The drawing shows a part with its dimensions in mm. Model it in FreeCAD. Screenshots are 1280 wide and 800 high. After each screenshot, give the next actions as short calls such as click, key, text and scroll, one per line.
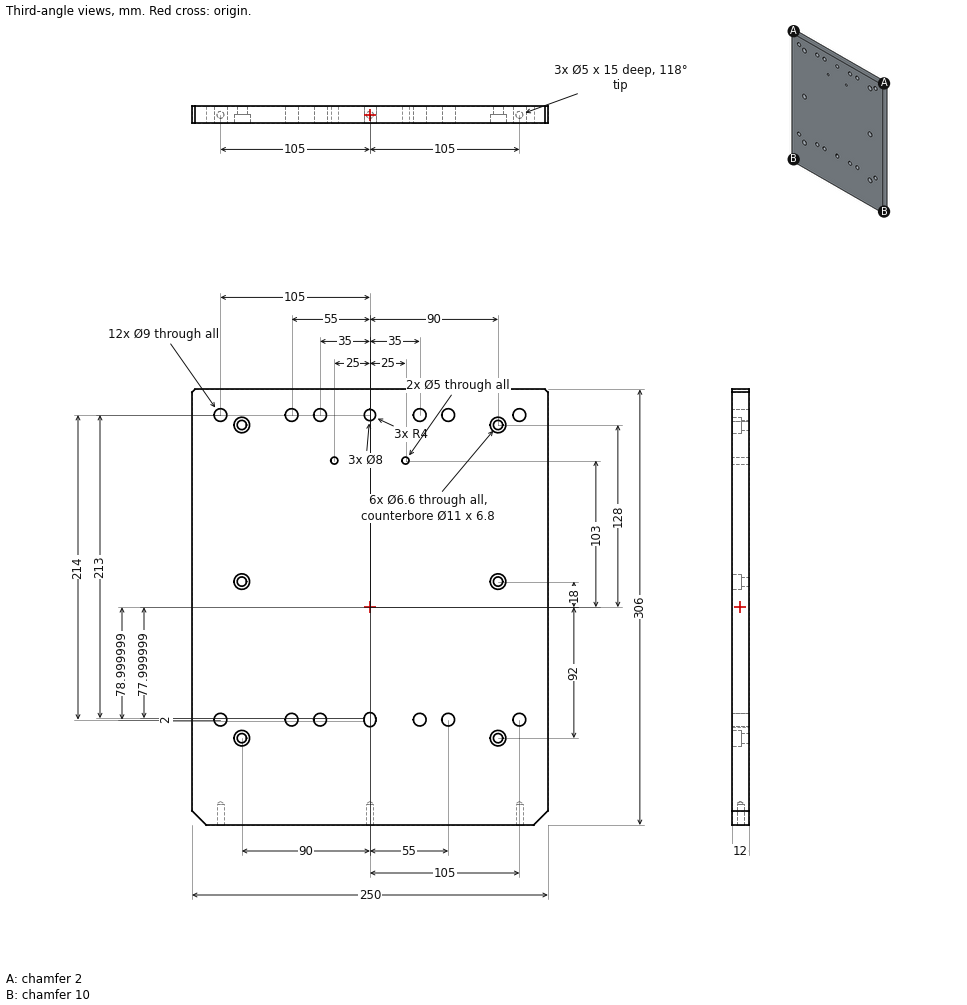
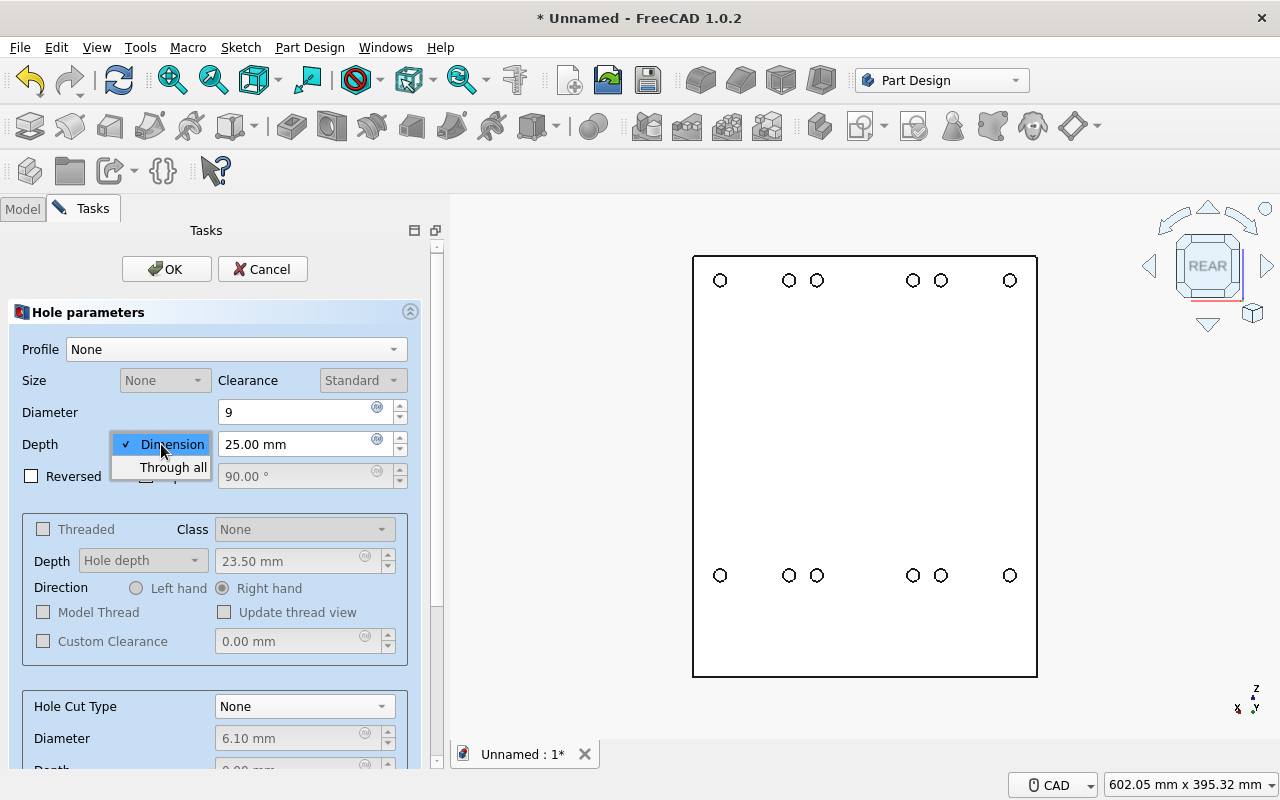
click(160, 468)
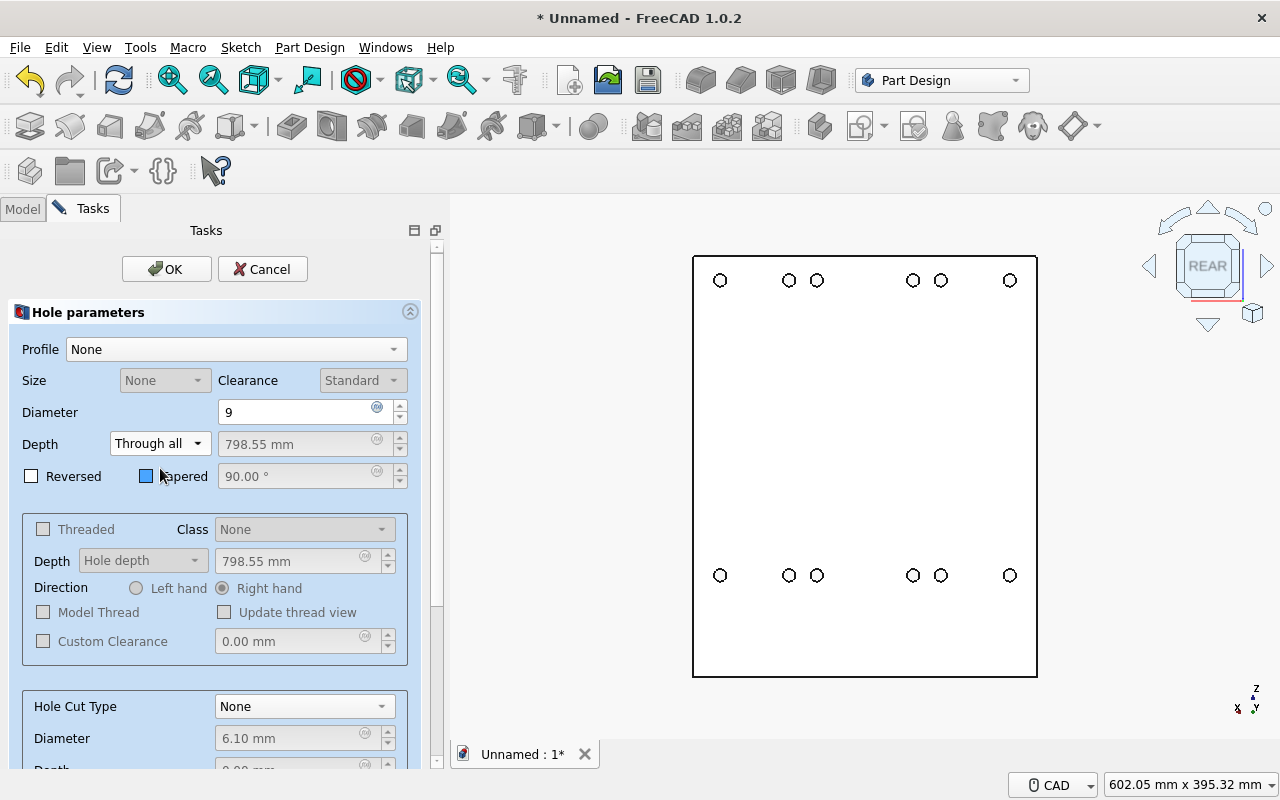
click(167, 269)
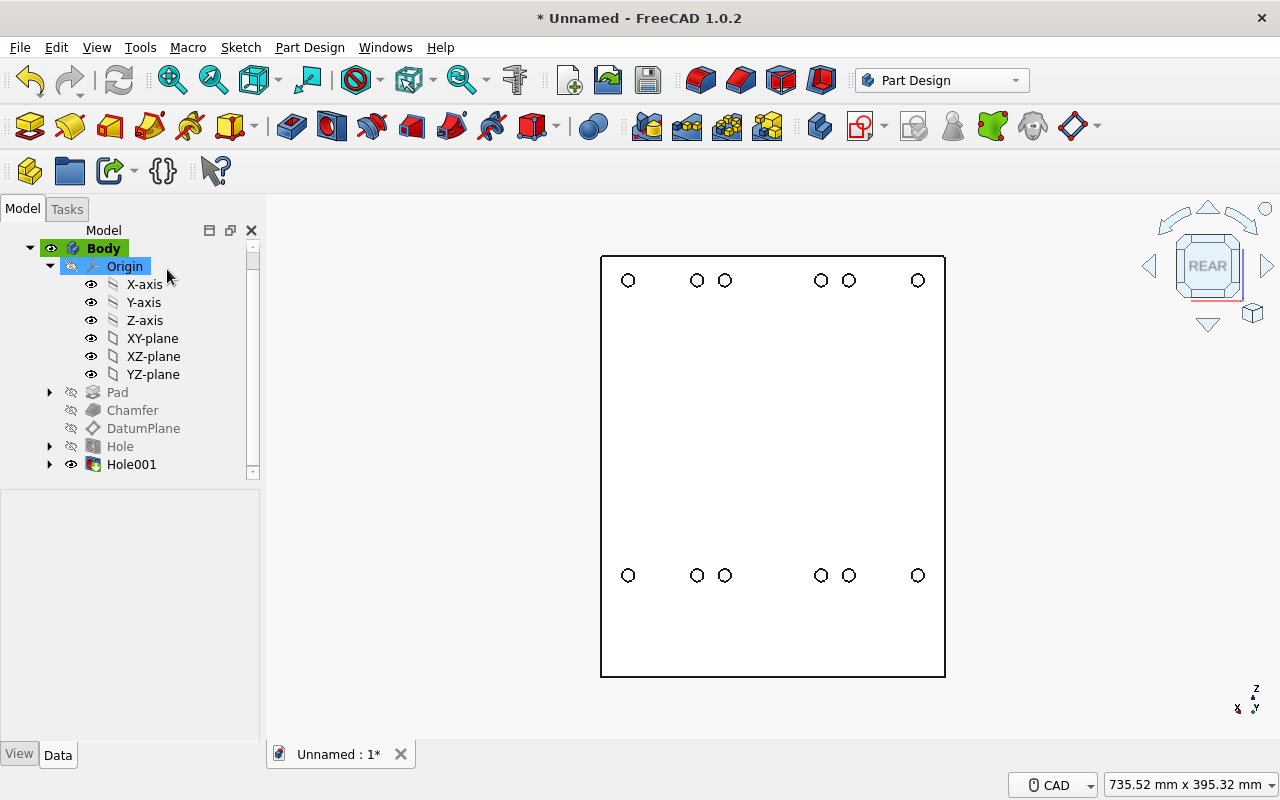
key(0)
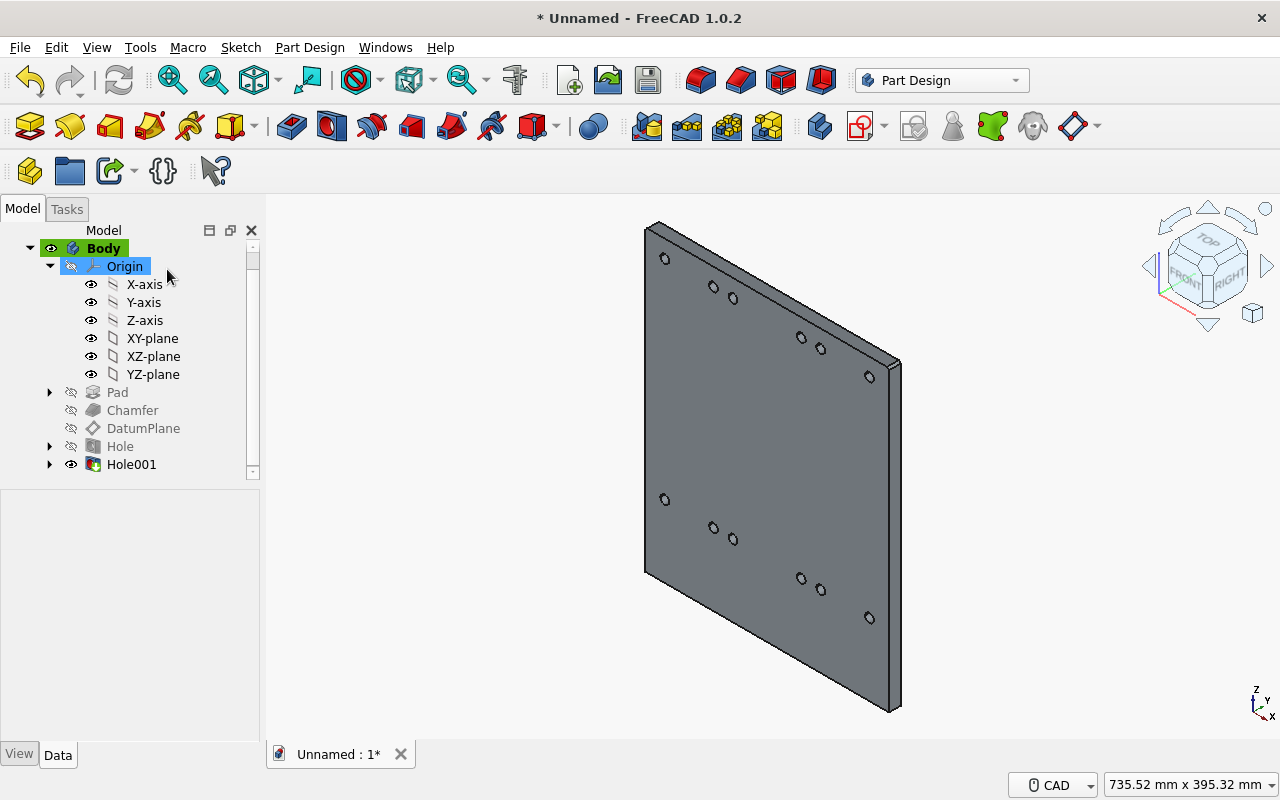
click(767, 420)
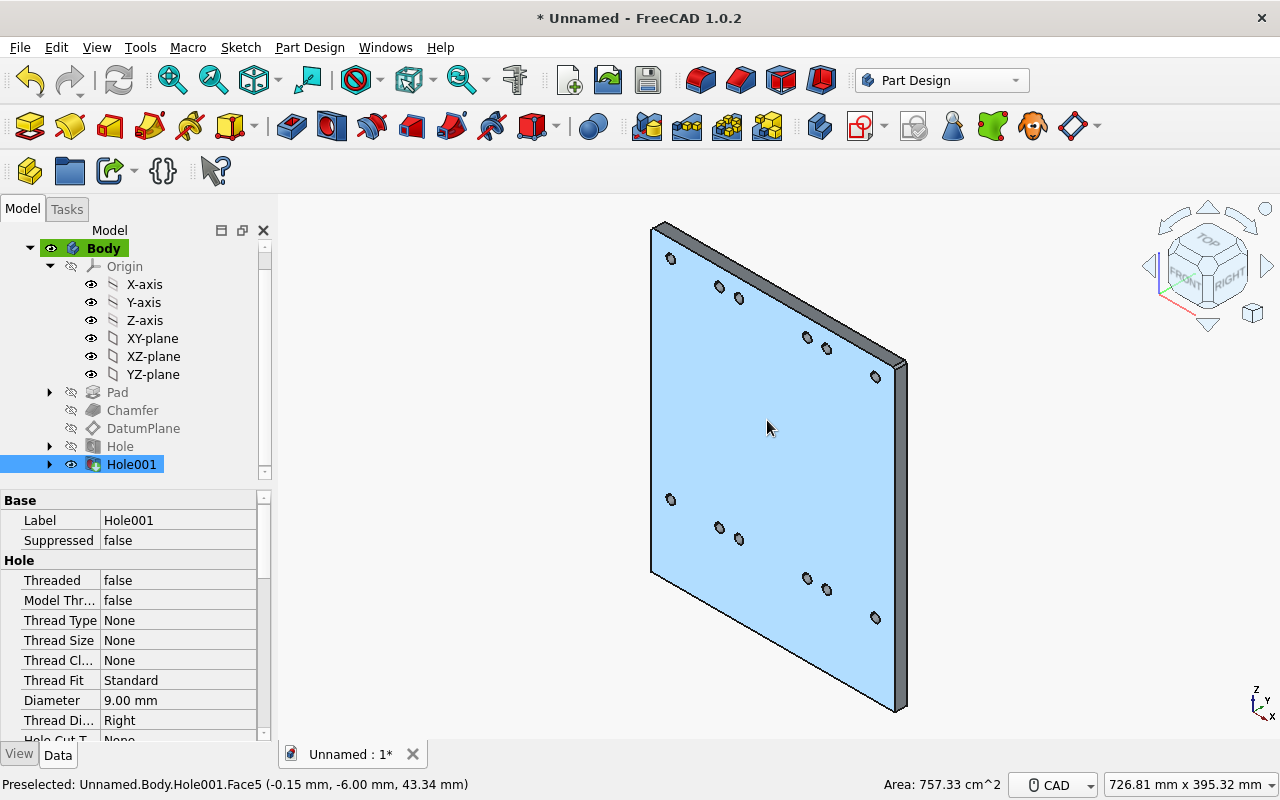
click(860, 126)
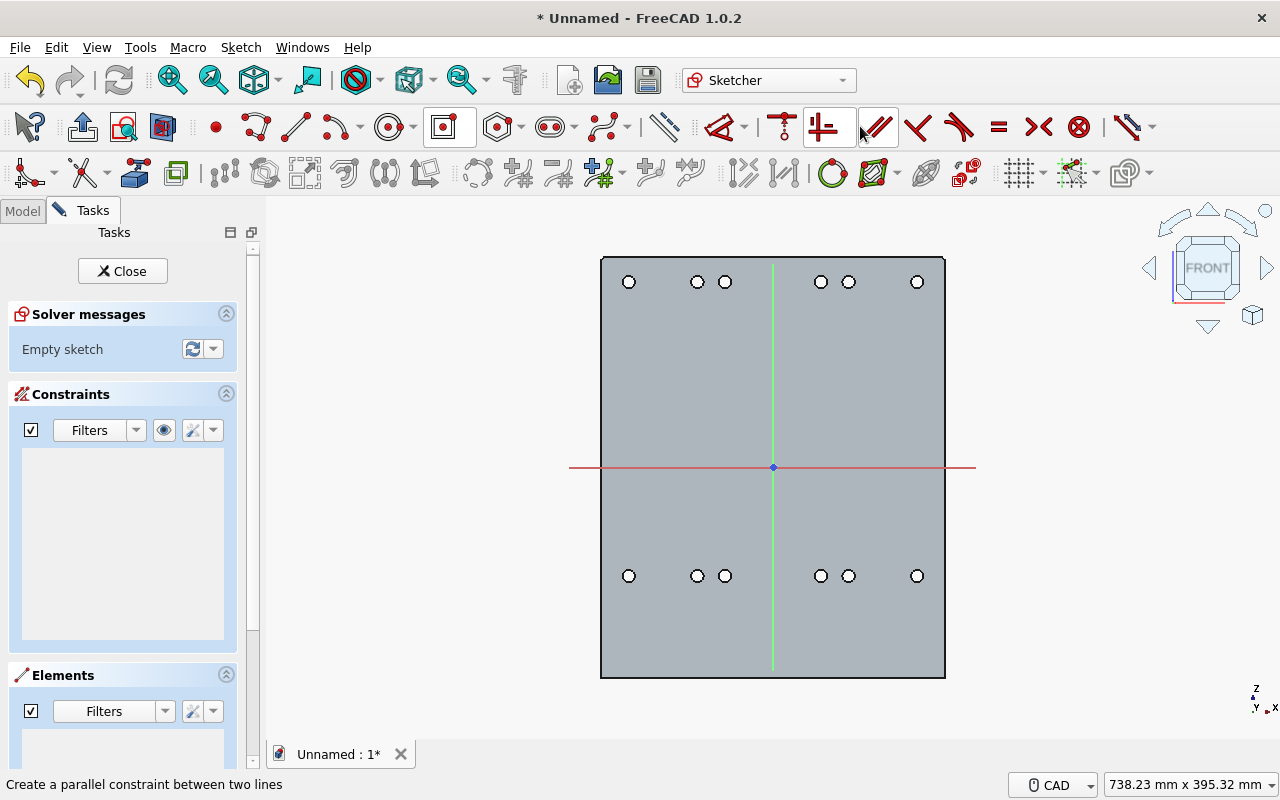
click(390, 128)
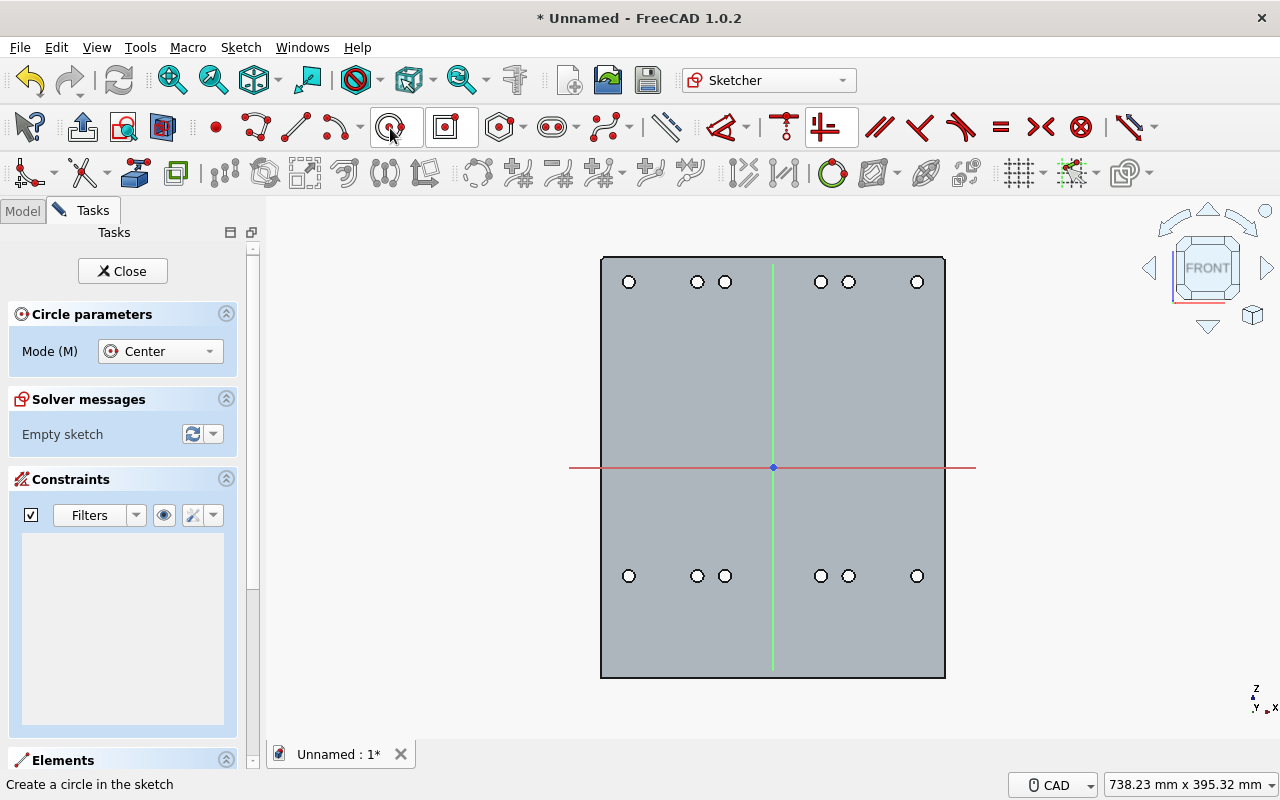
scroll(897, 292, up, 9)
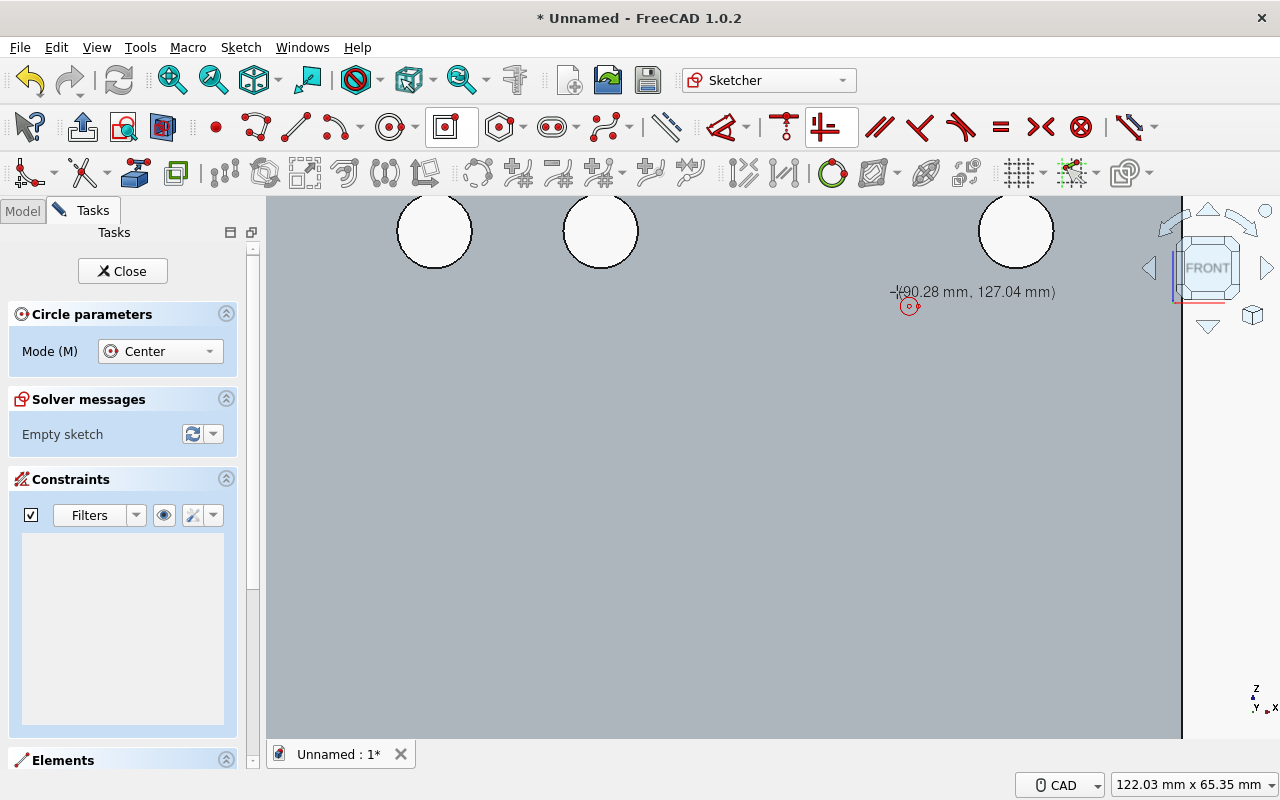
scroll(816, 322, down, 9)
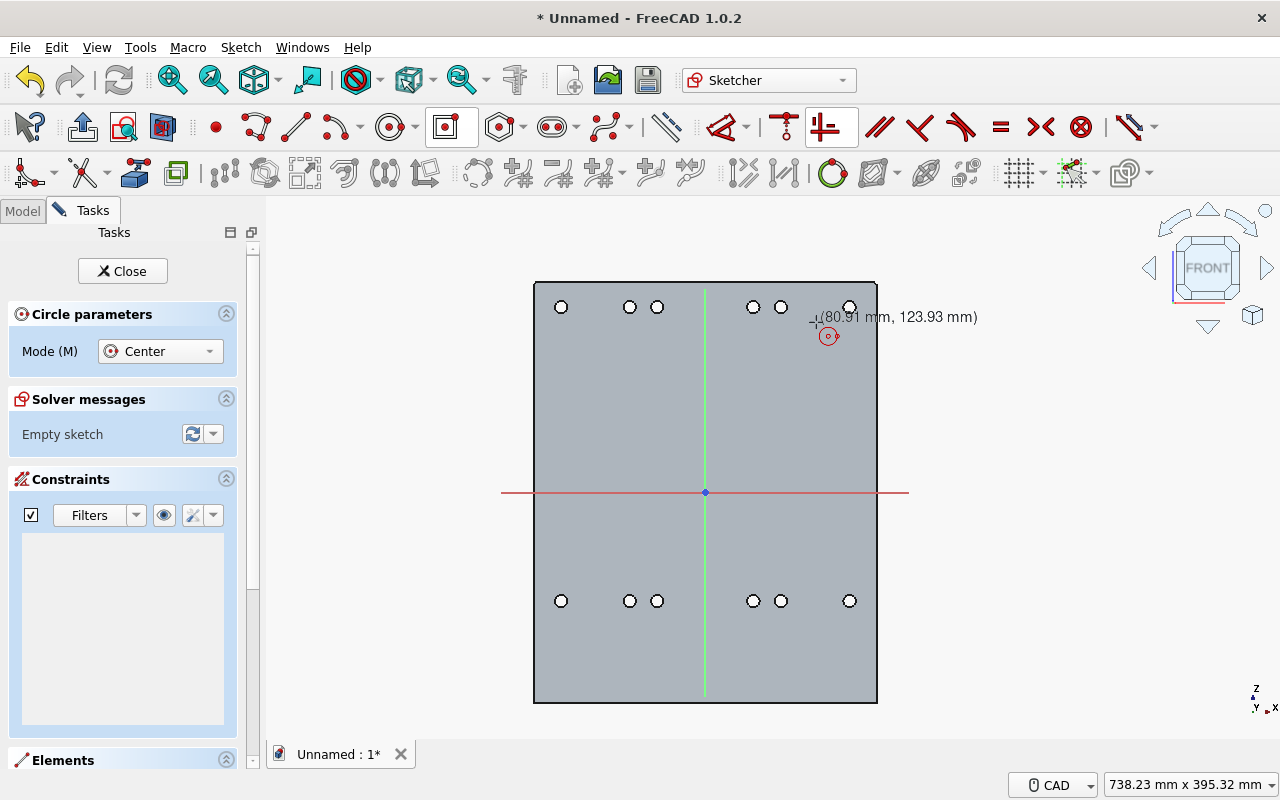
click(829, 317)
move(832, 314)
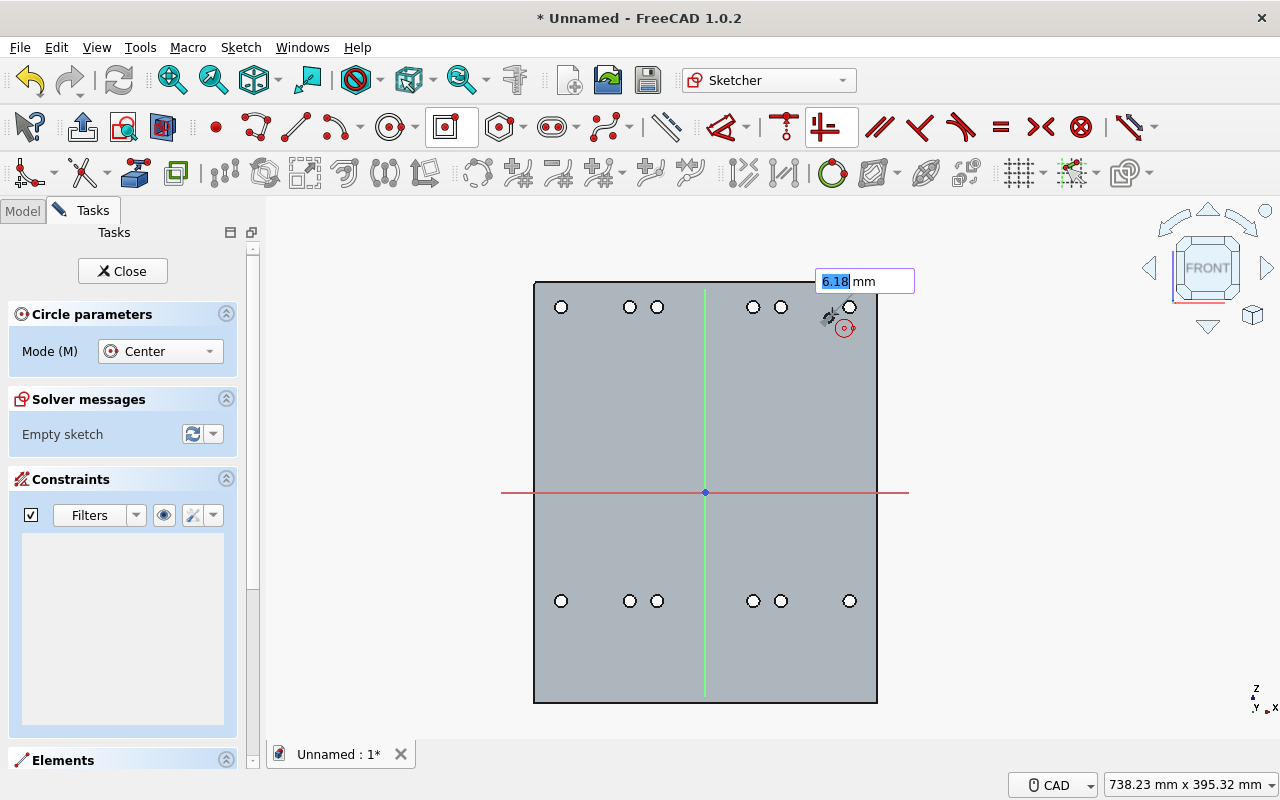
text(6.6)
key(Return)